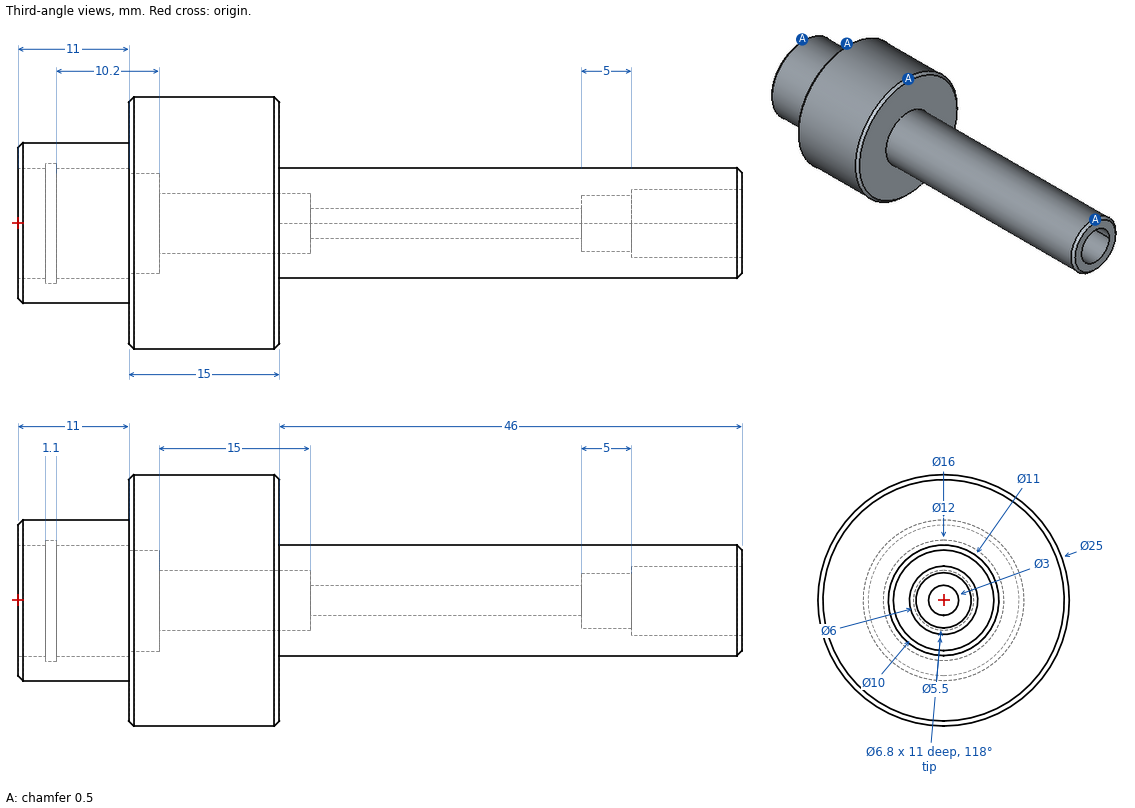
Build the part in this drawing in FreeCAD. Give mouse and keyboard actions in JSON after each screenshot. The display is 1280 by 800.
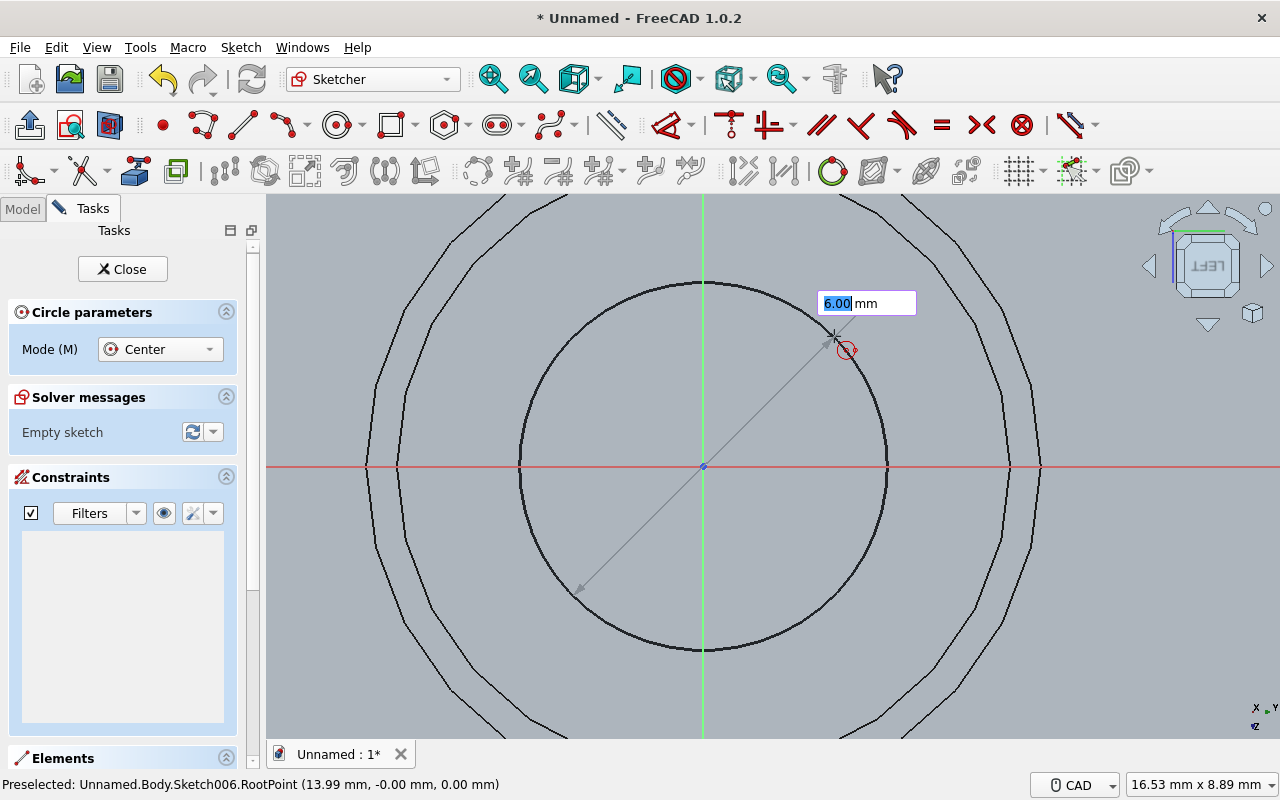
{"action": "type", "text": "6"}
{"action": "key", "text": "Return"}
{"action": "key", "text": "Escape"}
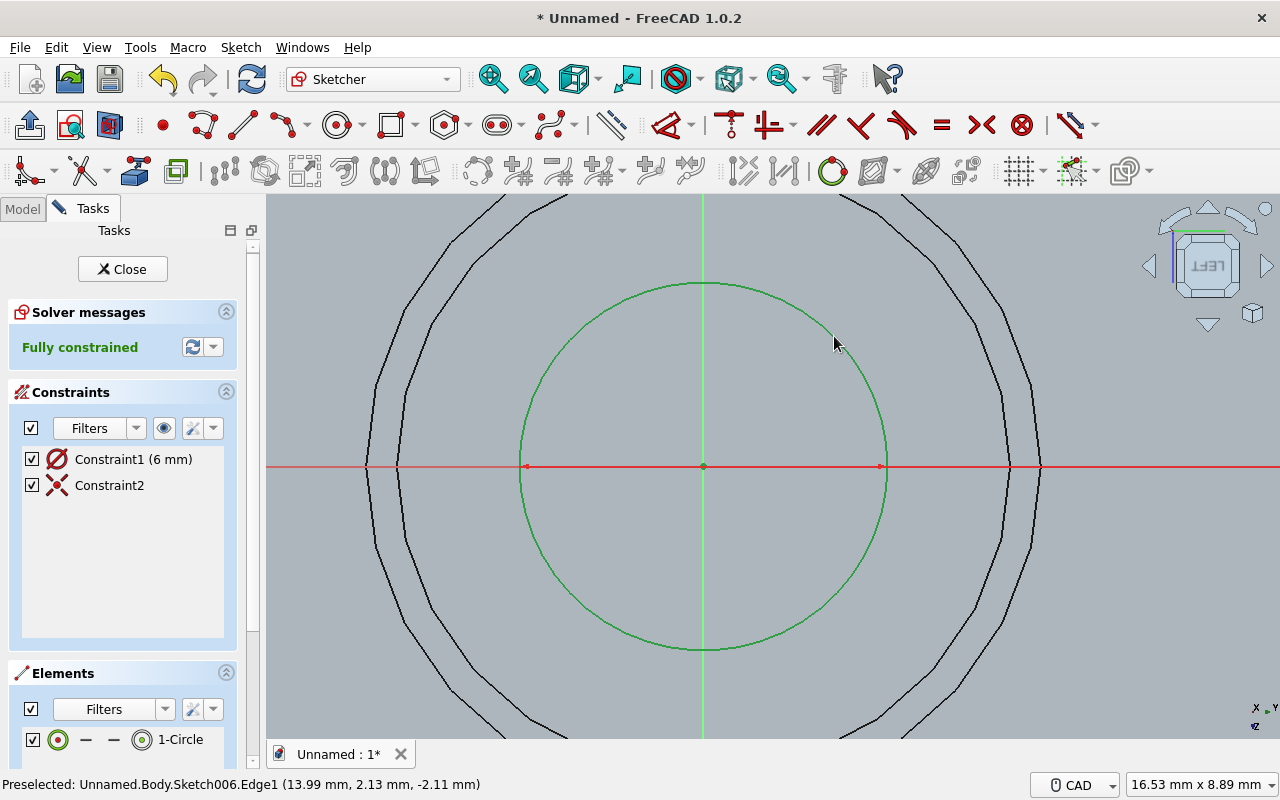
{"action": "left_click", "coordinate": [123, 269]}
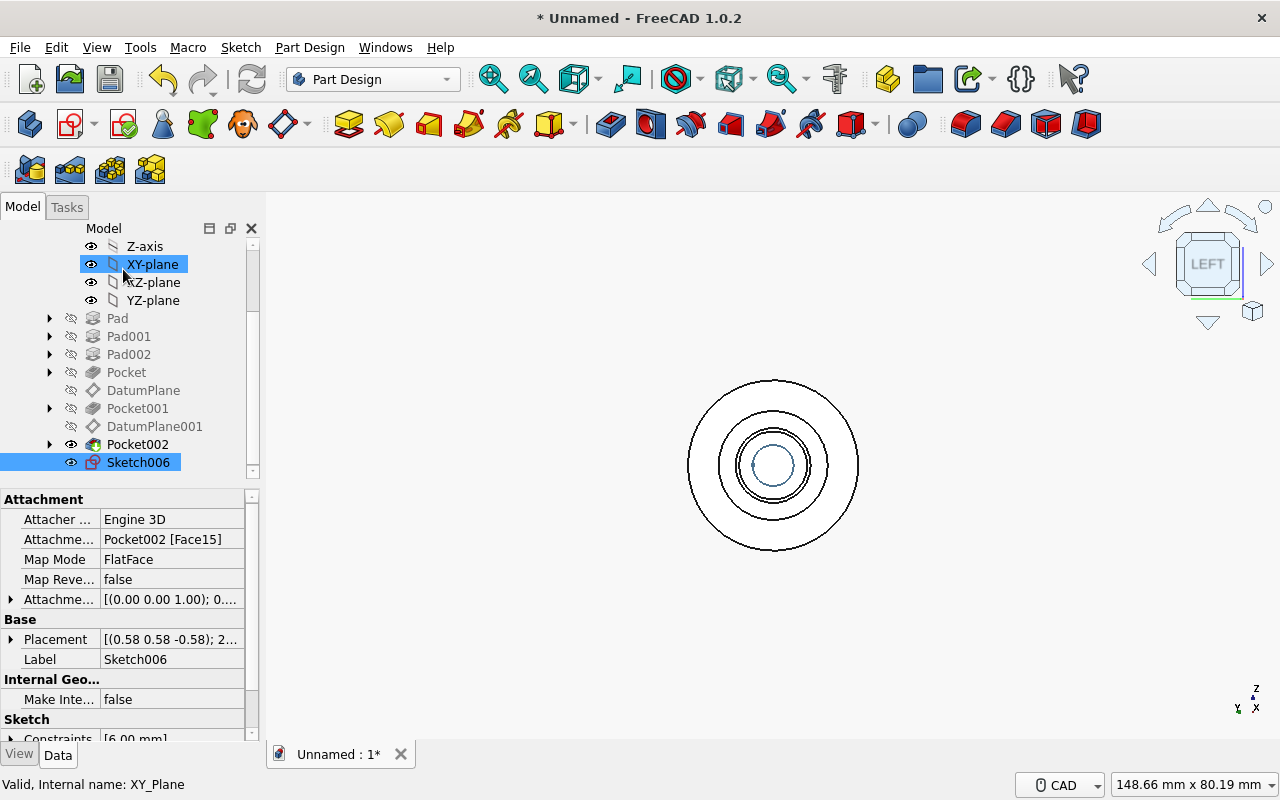
{"action": "left_click", "coordinate": [612, 124]}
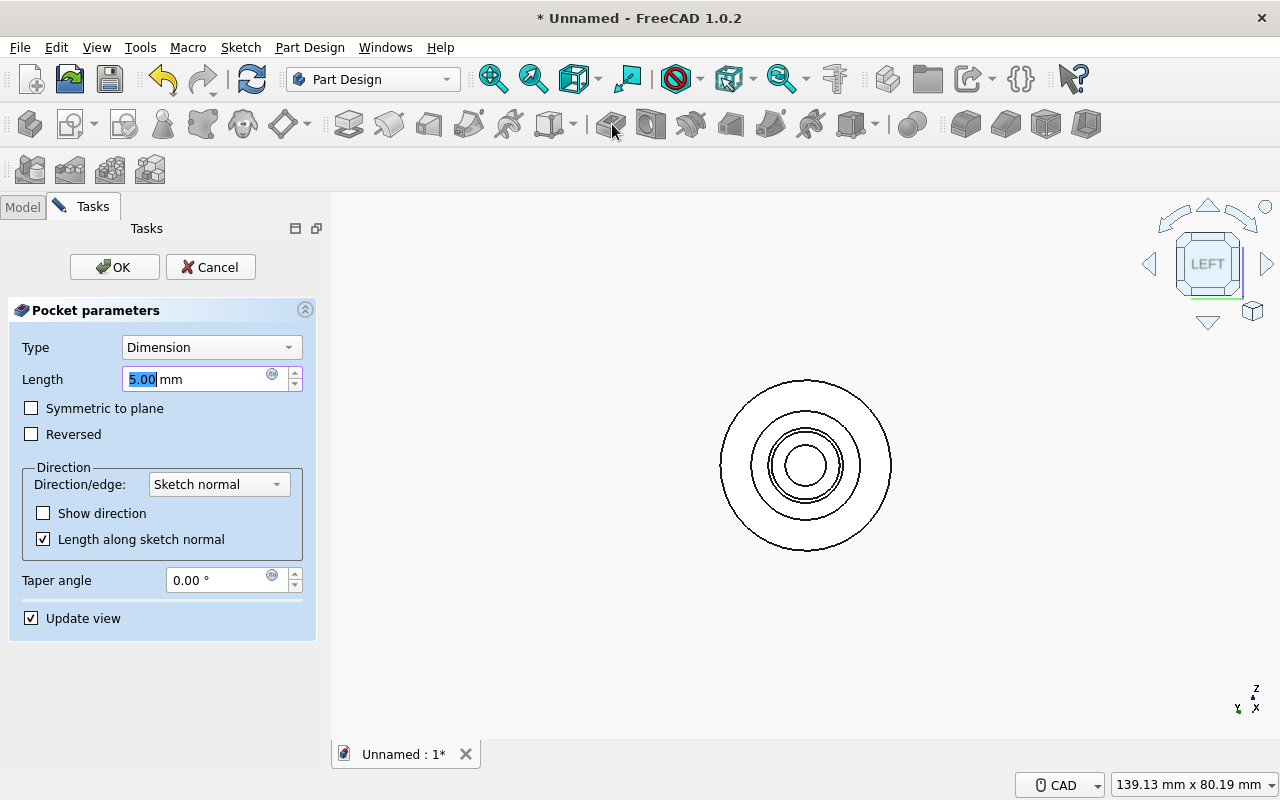
{"action": "type", "text": "15"}
{"action": "key", "text": "Tab"}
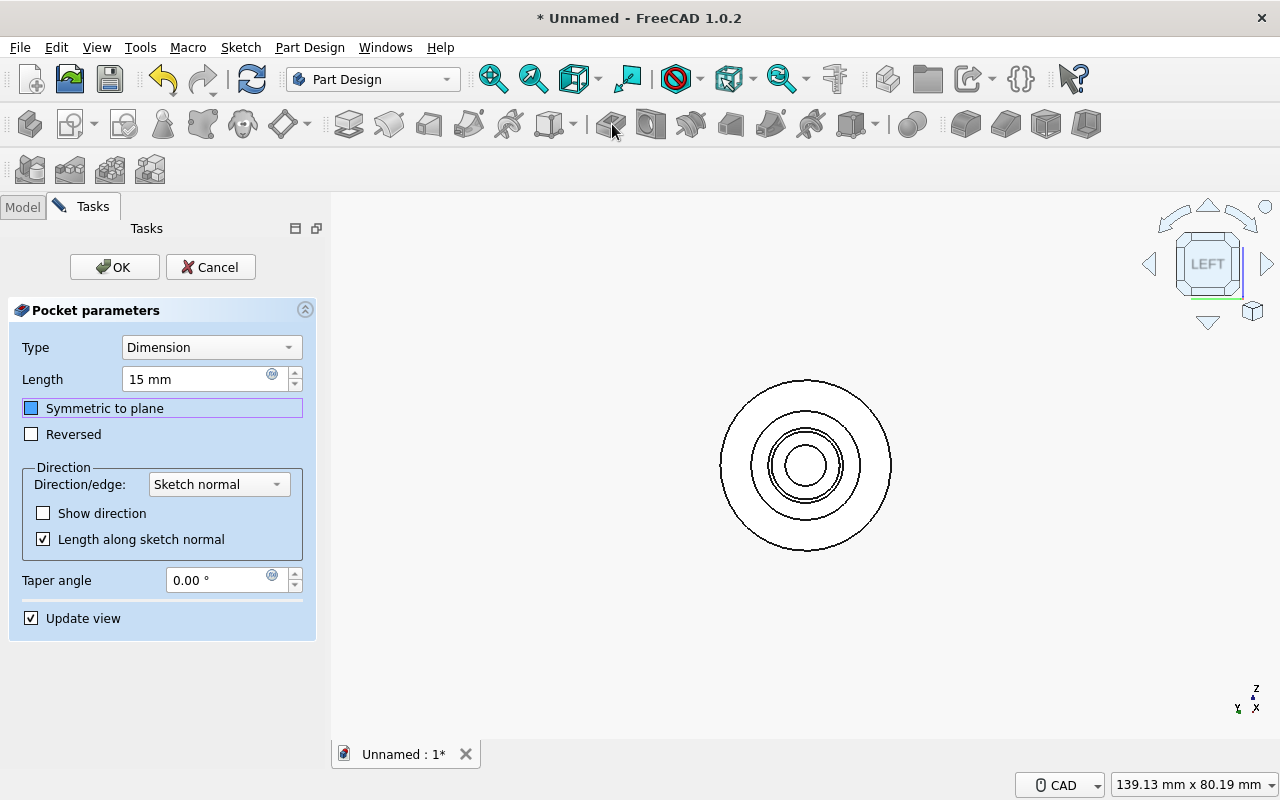
{"action": "left_click", "coordinate": [115, 267]}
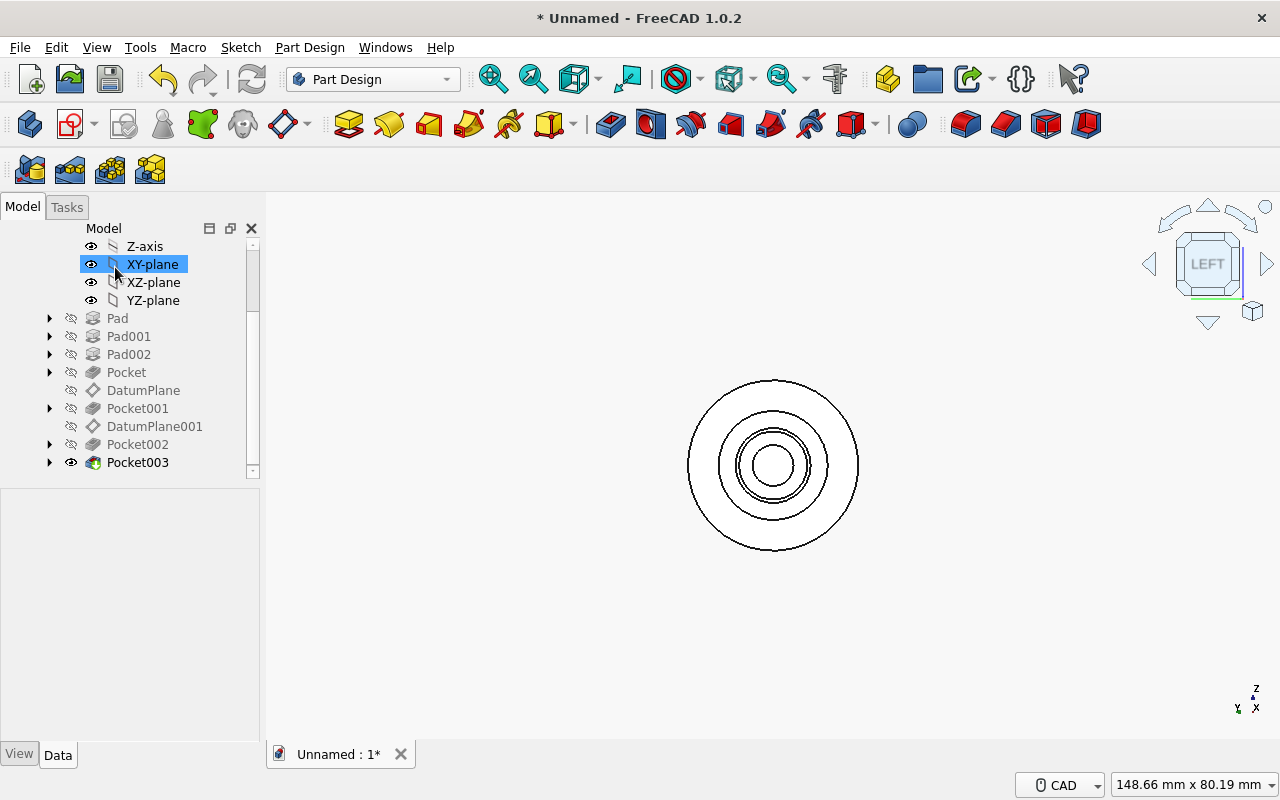
{"action": "left_click", "coordinate": [494, 80]}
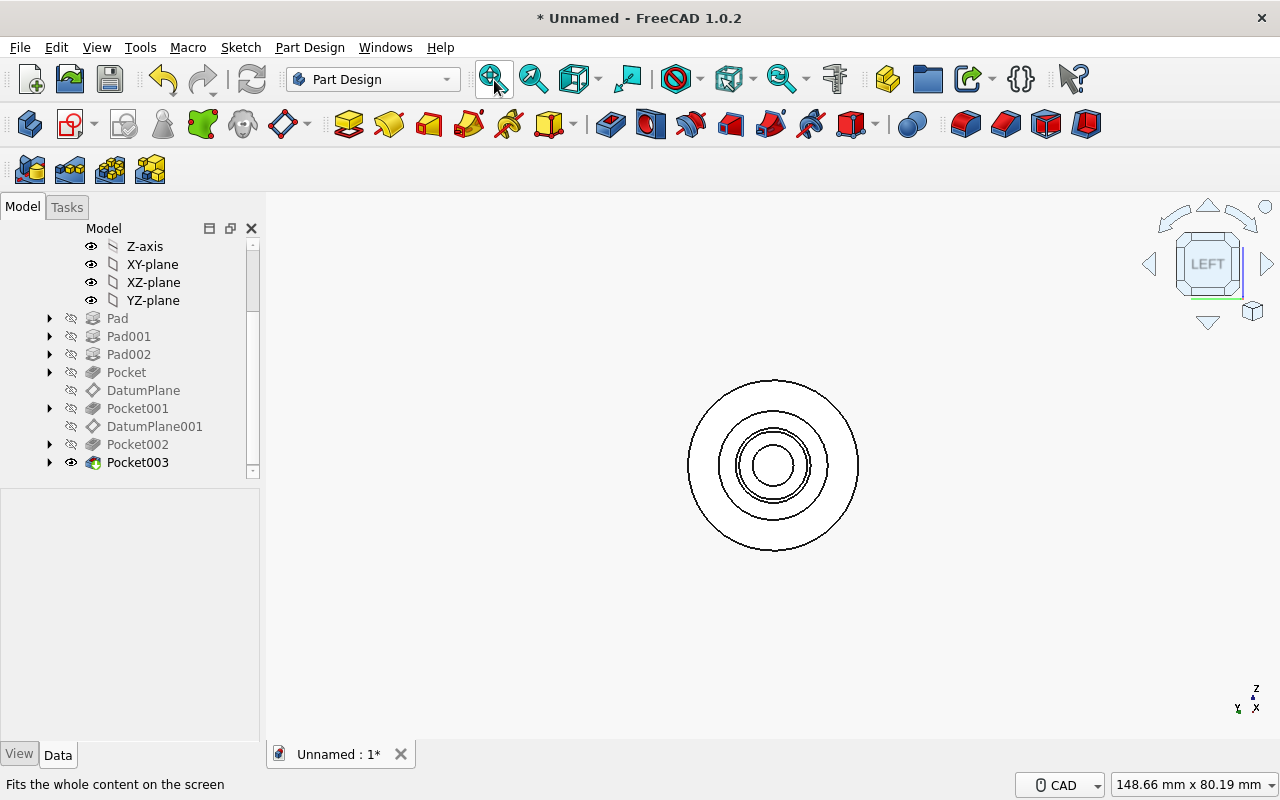
{"action": "key", "text": "0"}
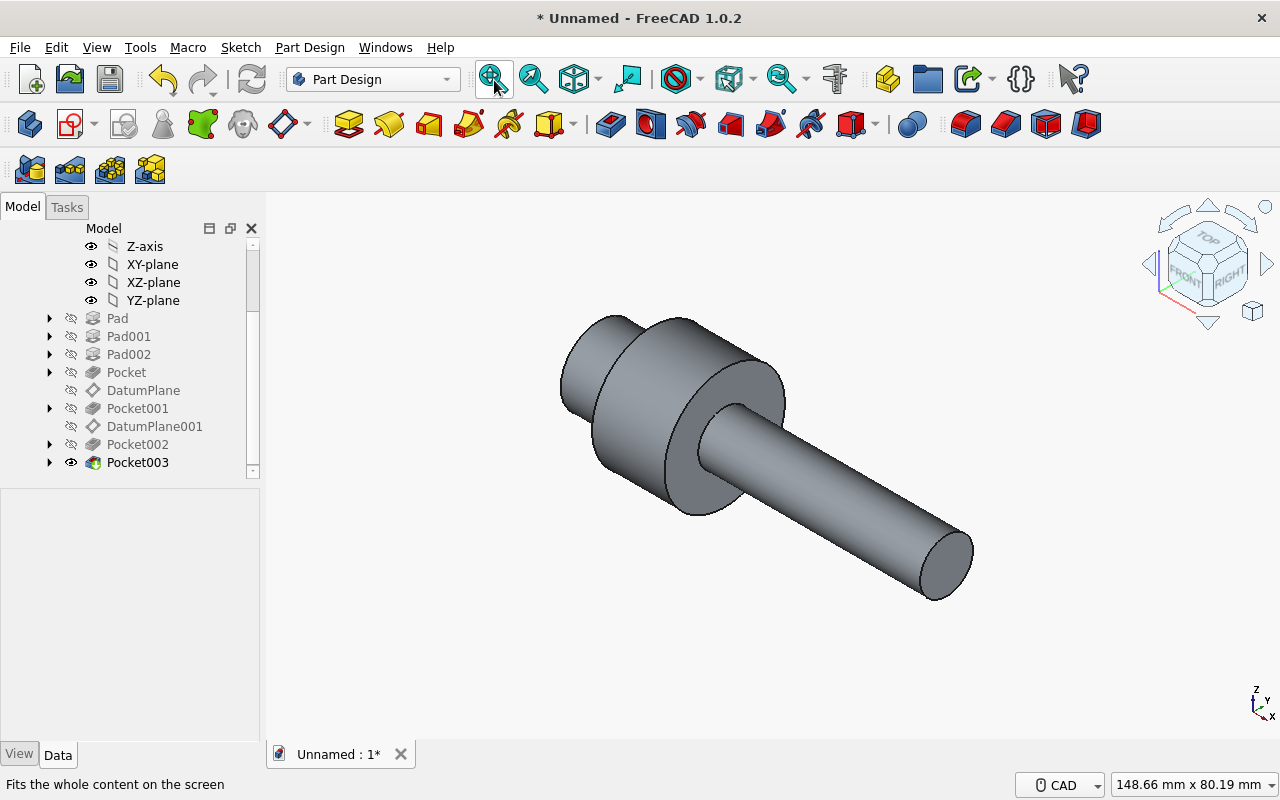
{"action": "left_click", "coordinate": [947, 565]}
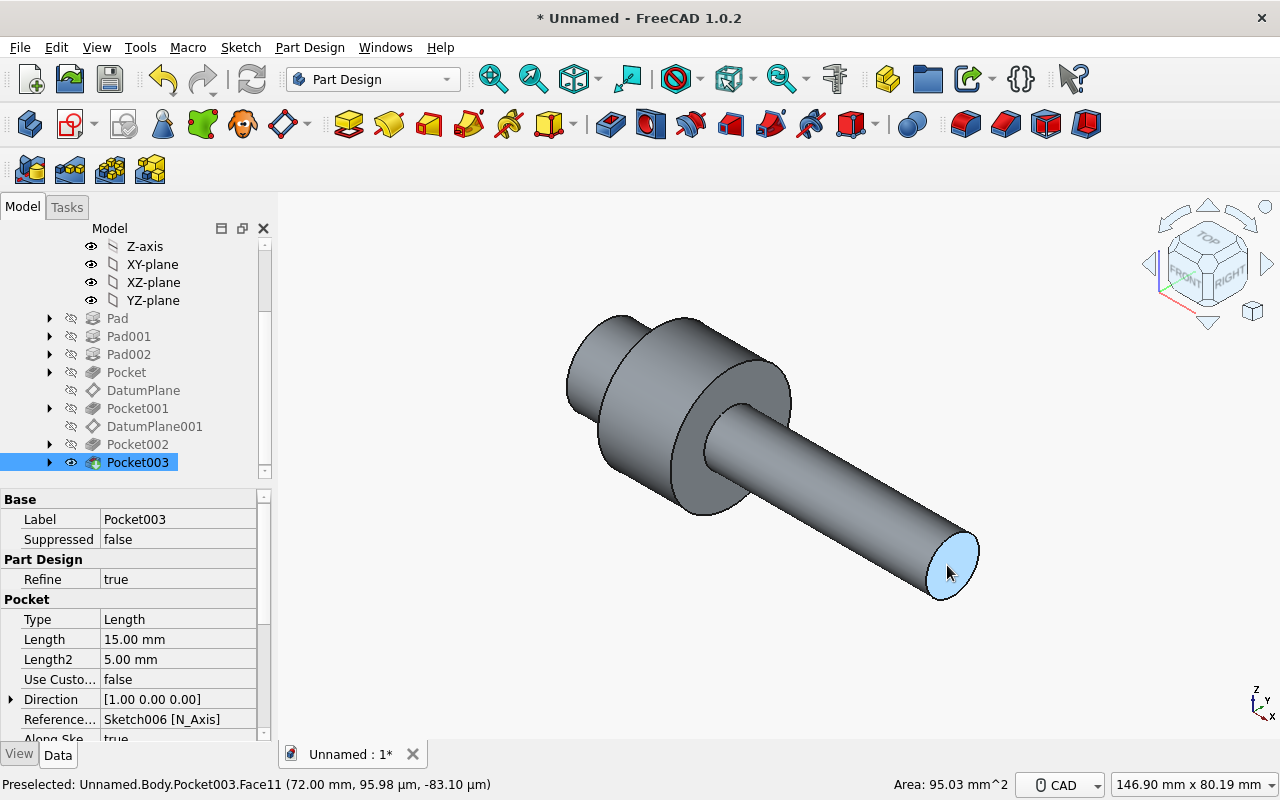
{"action": "left_click", "coordinate": [70, 124]}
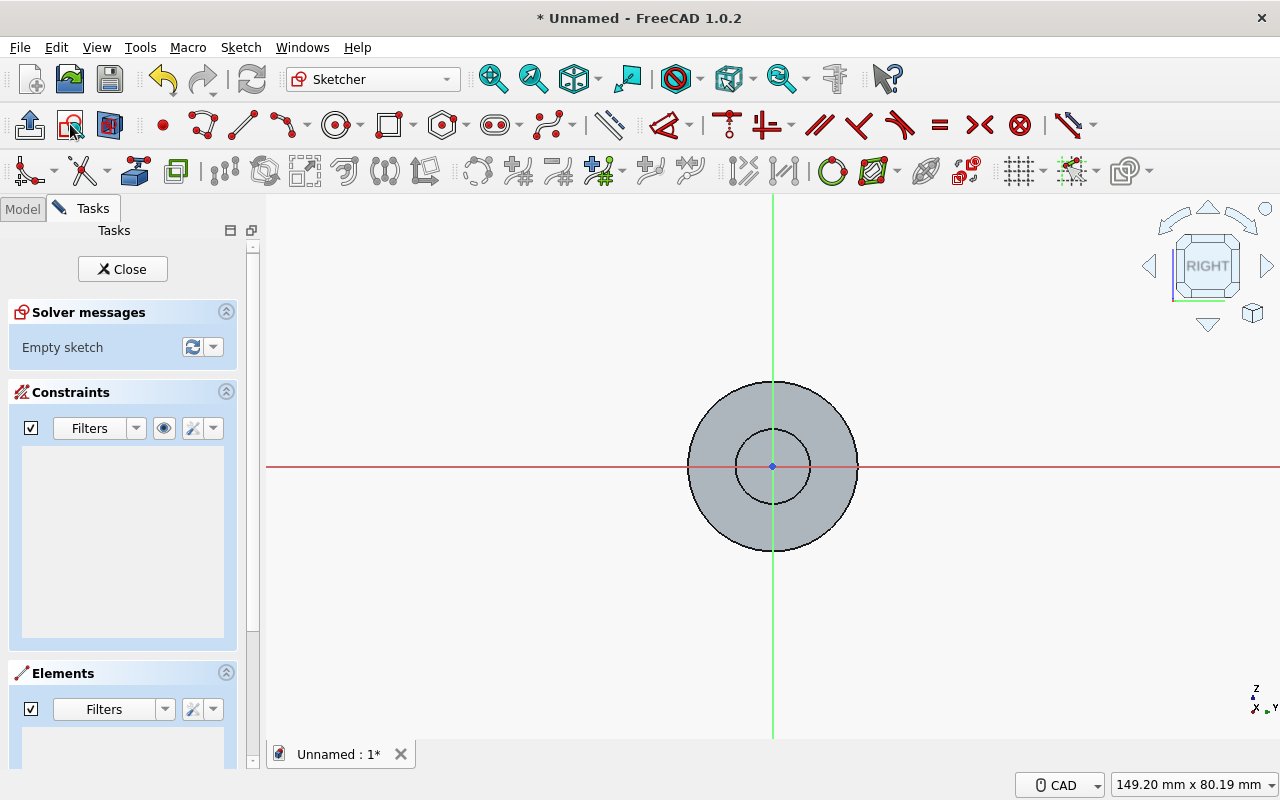
{"action": "scroll", "coordinate": [784, 466], "scroll_direction": "up", "scroll_amount": 10}